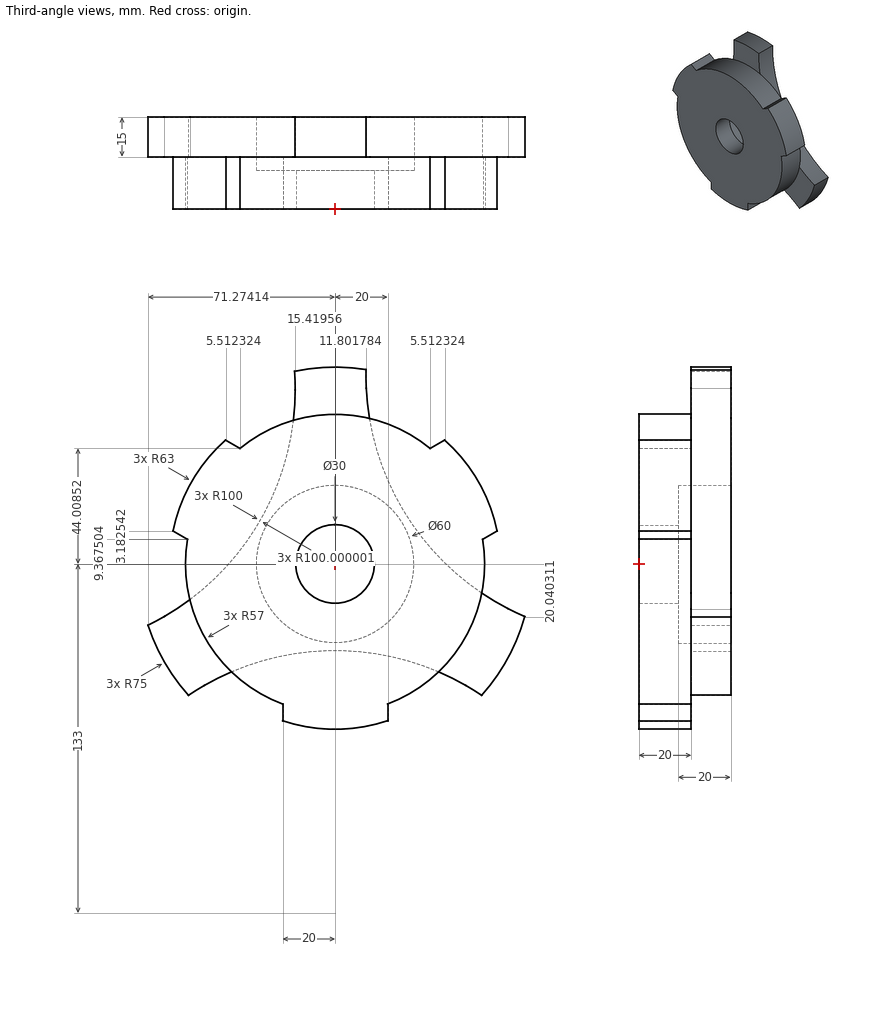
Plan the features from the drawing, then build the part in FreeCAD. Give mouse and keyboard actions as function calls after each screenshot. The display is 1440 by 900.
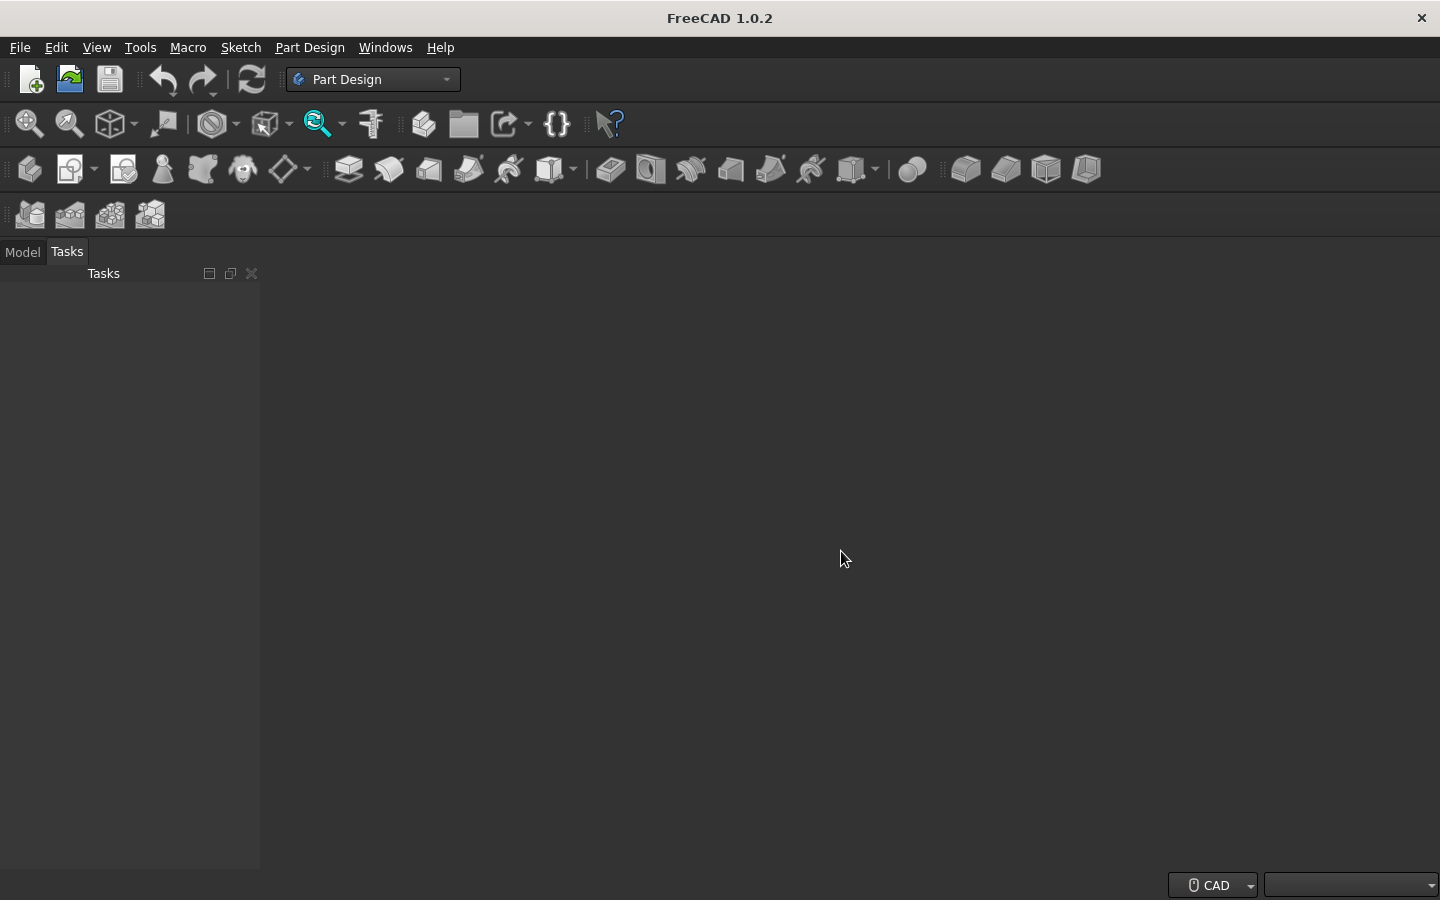
click(30, 80)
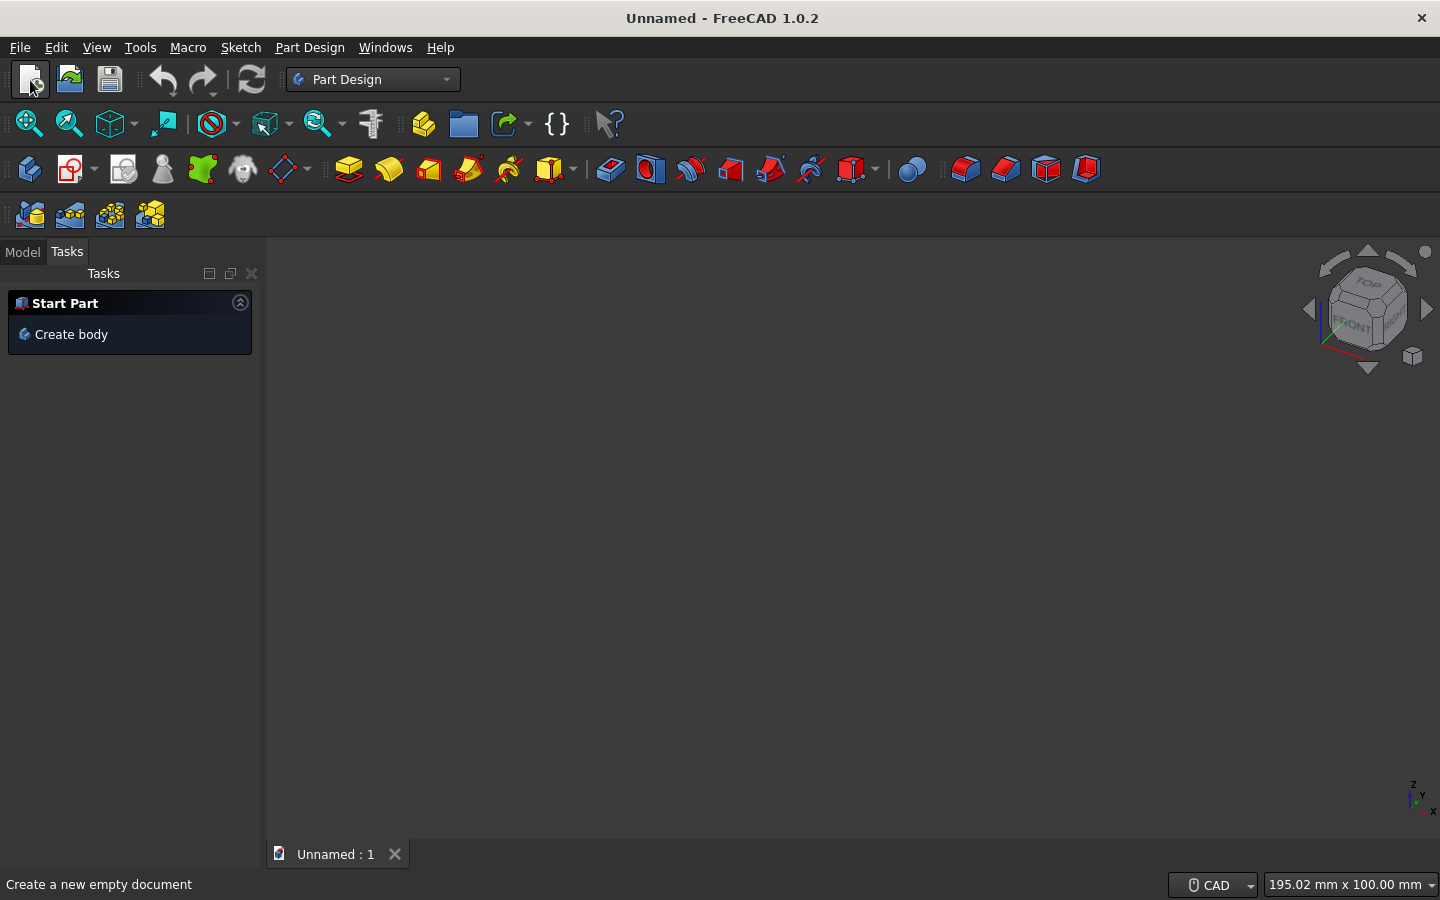
click(70, 170)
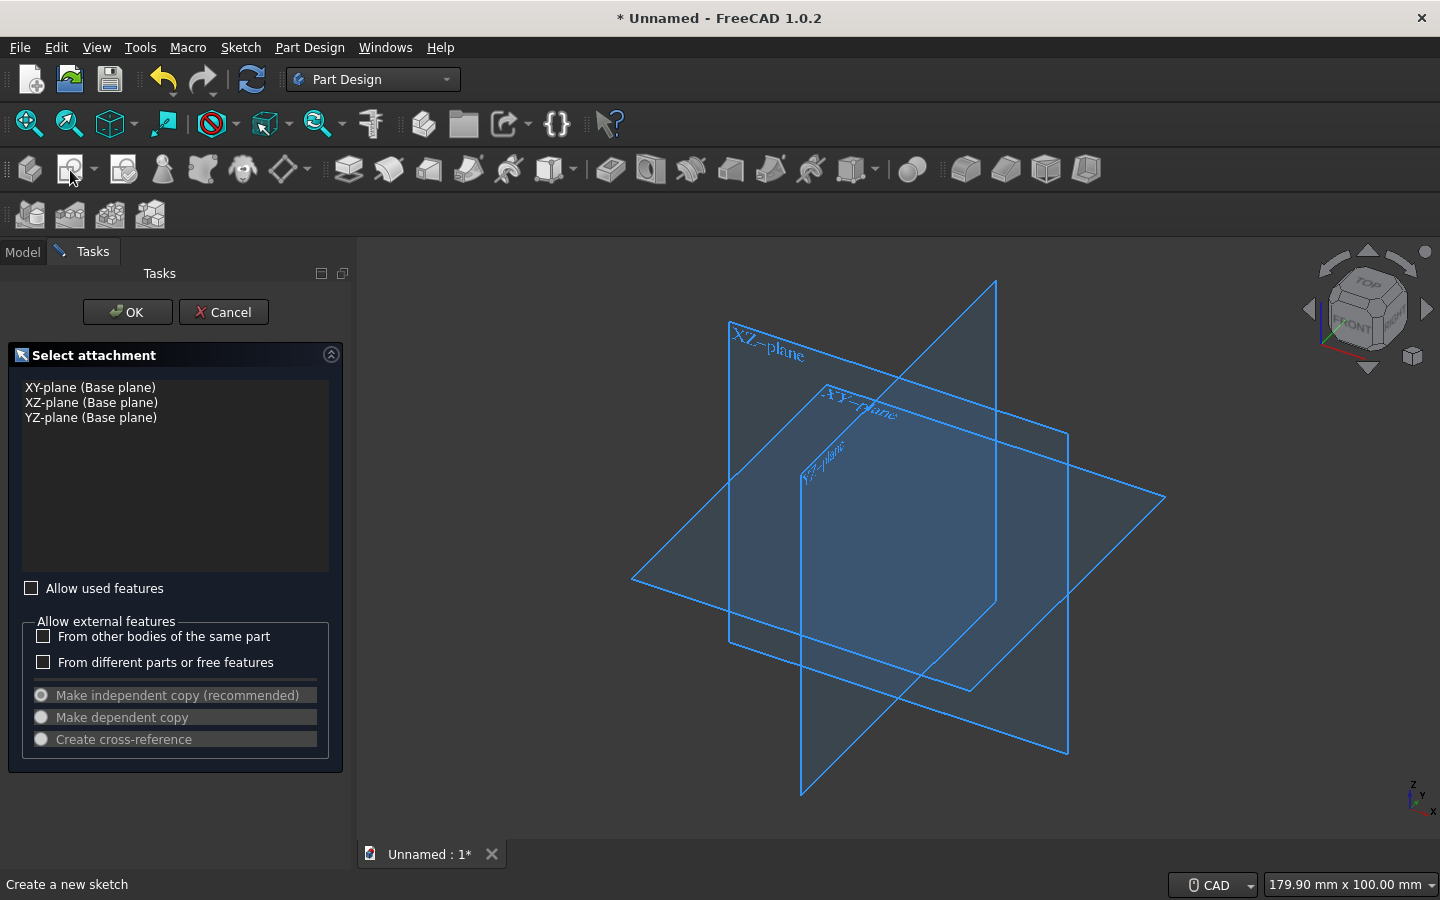
click(82, 402)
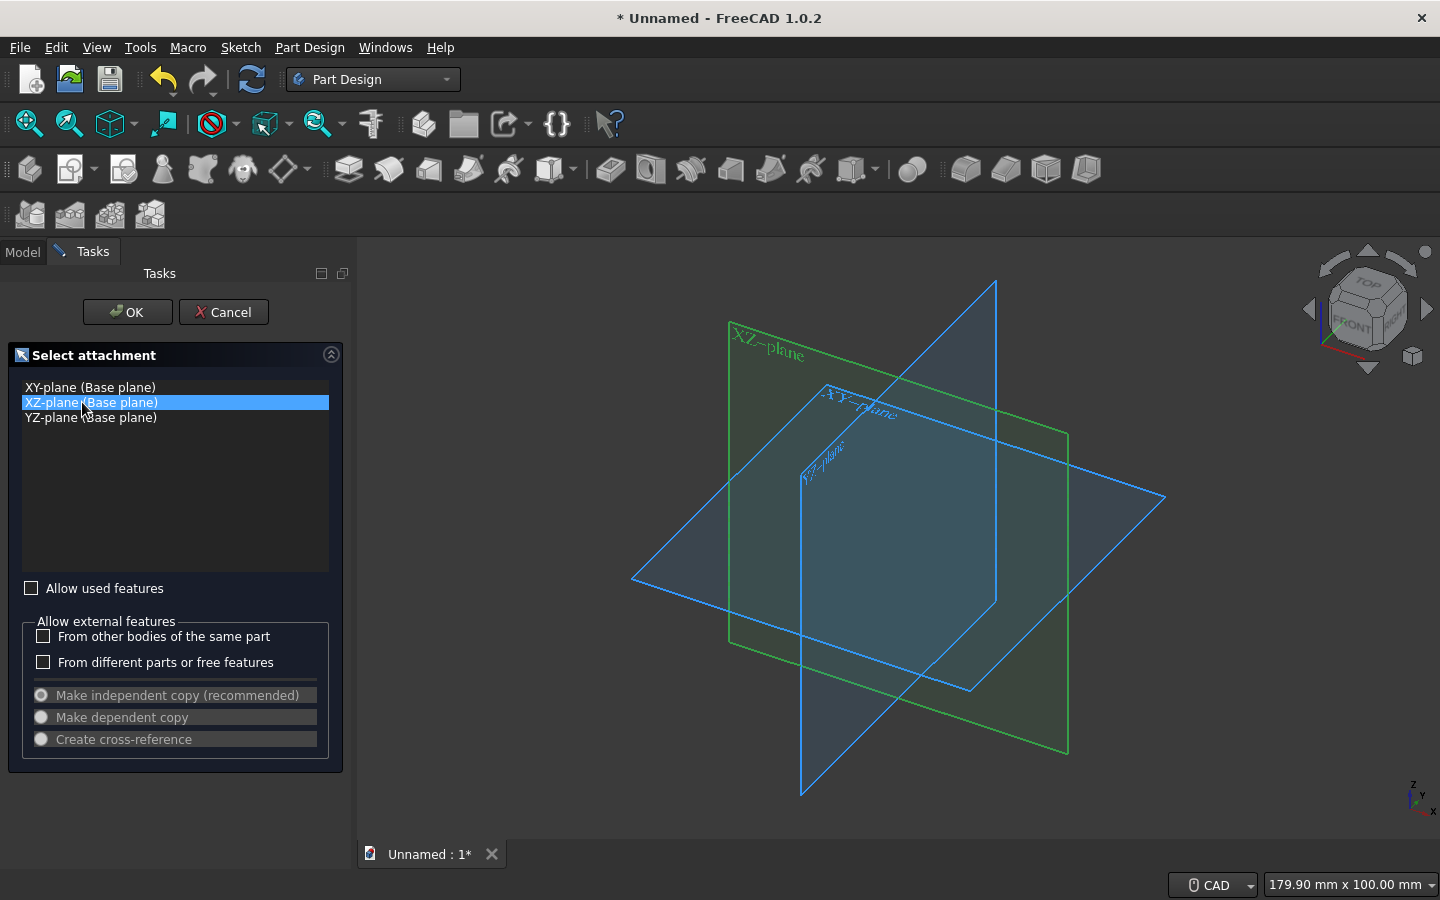
click(128, 312)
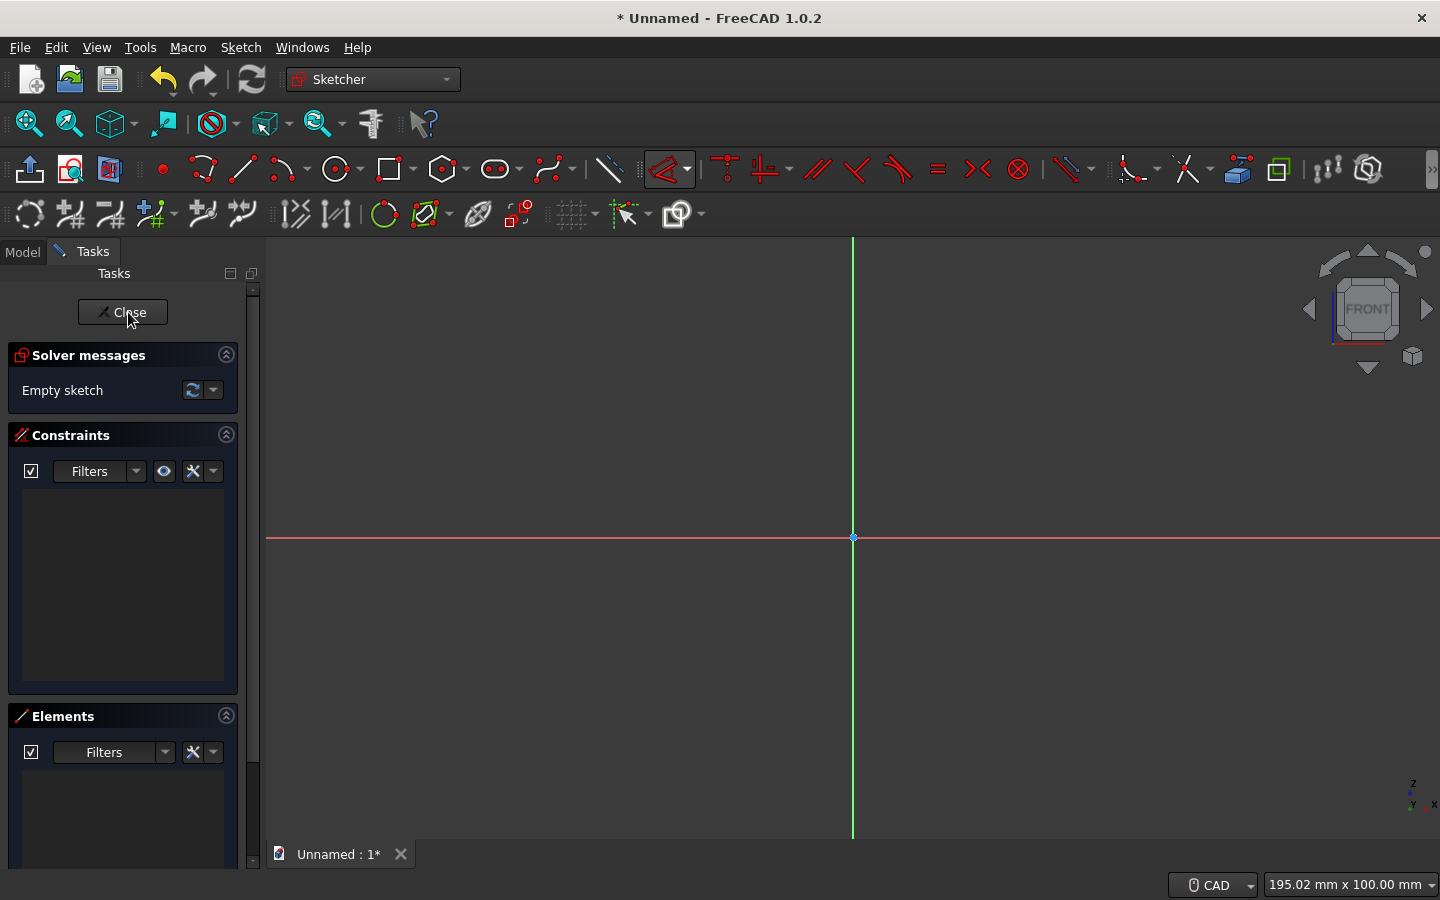
scroll(701, 516, down, 3)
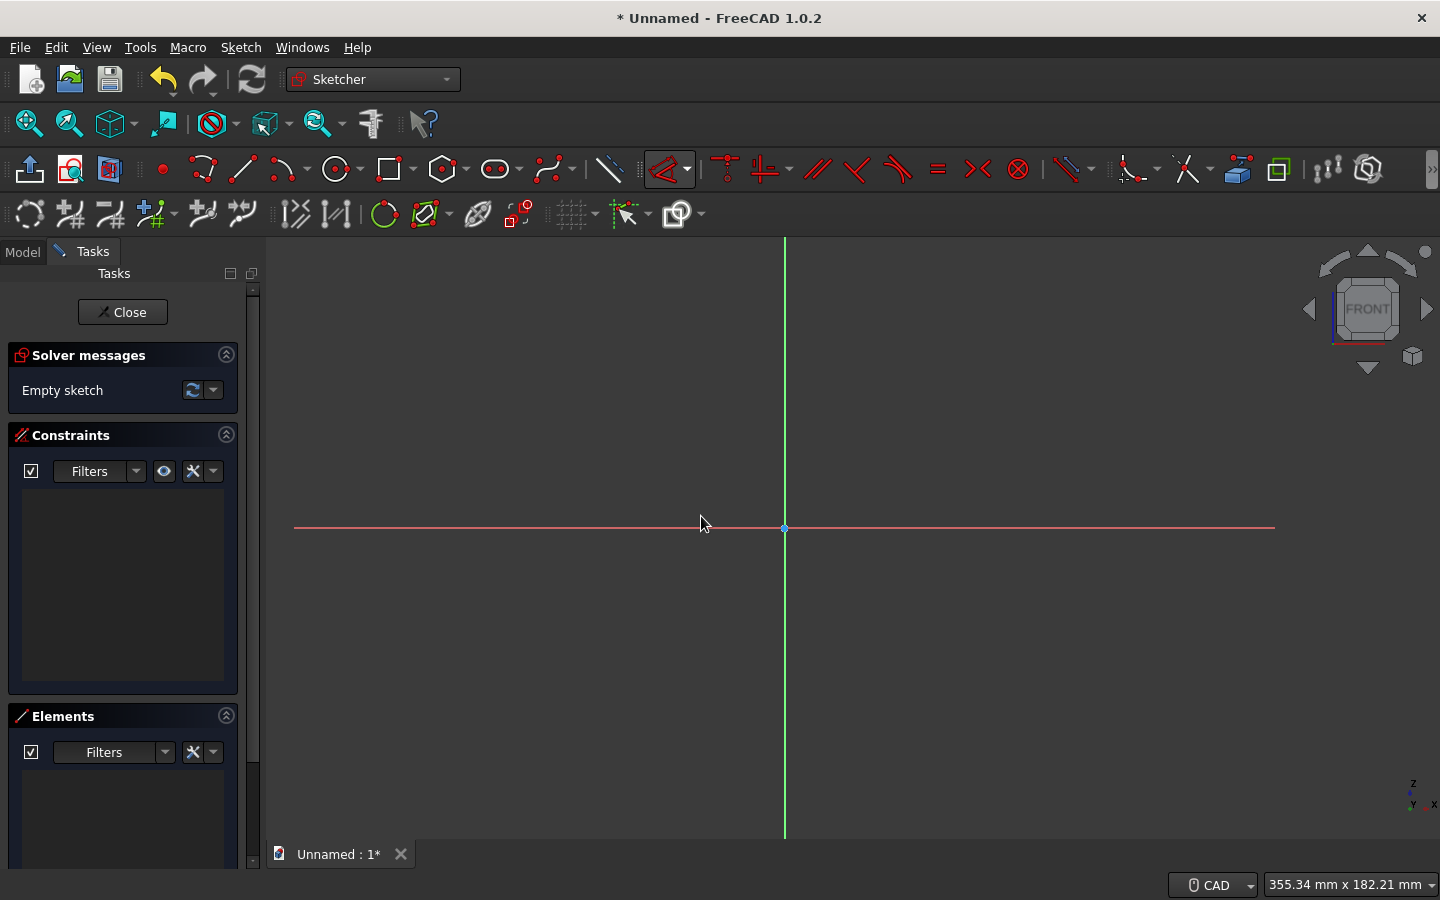
click(244, 170)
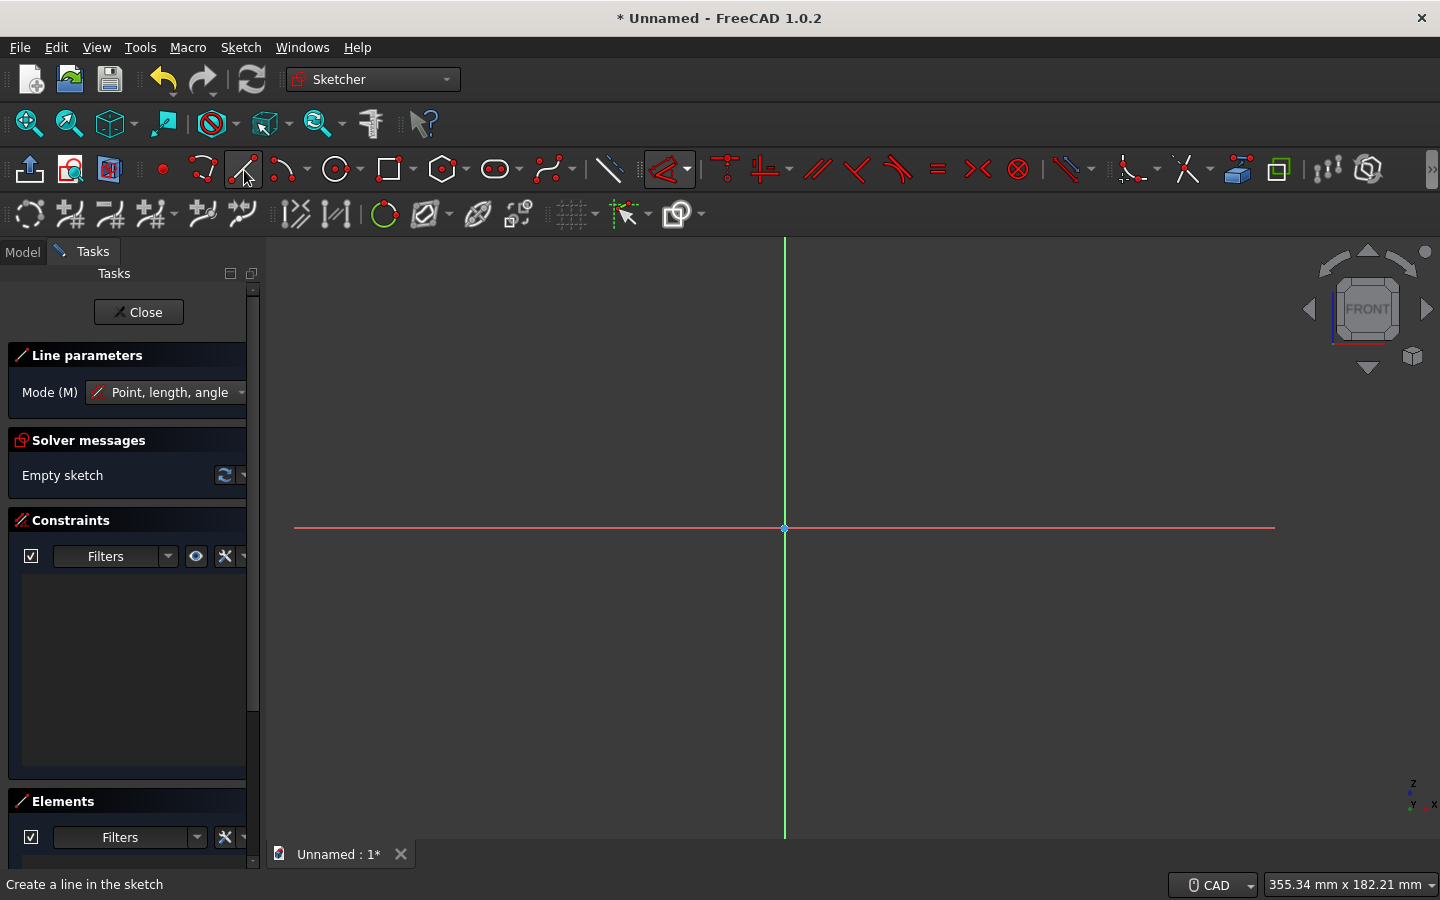
click(719, 726)
click(719, 705)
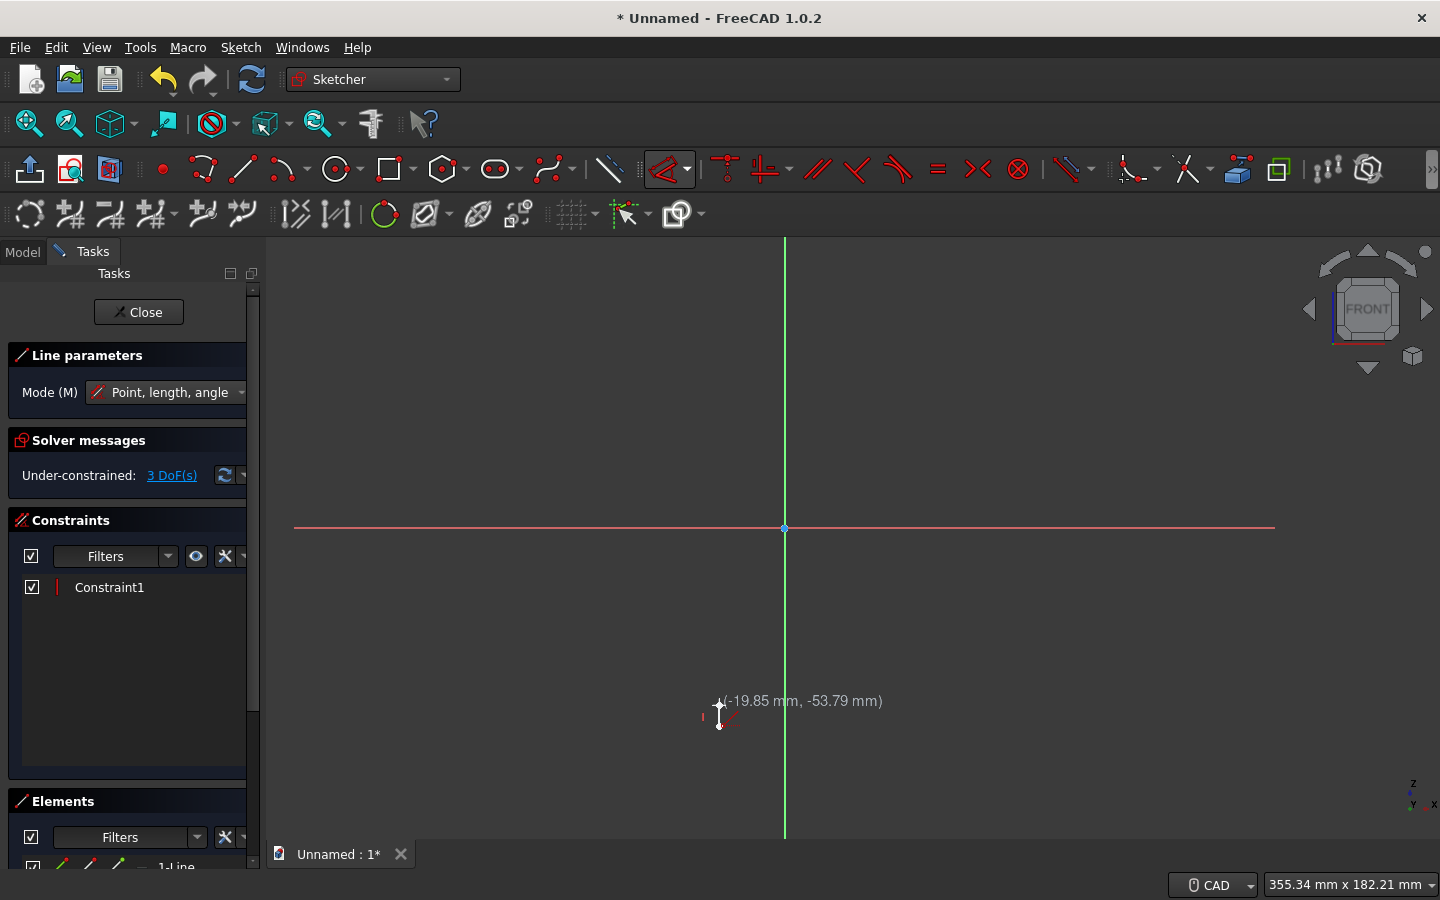
click(599, 497)
click(581, 487)